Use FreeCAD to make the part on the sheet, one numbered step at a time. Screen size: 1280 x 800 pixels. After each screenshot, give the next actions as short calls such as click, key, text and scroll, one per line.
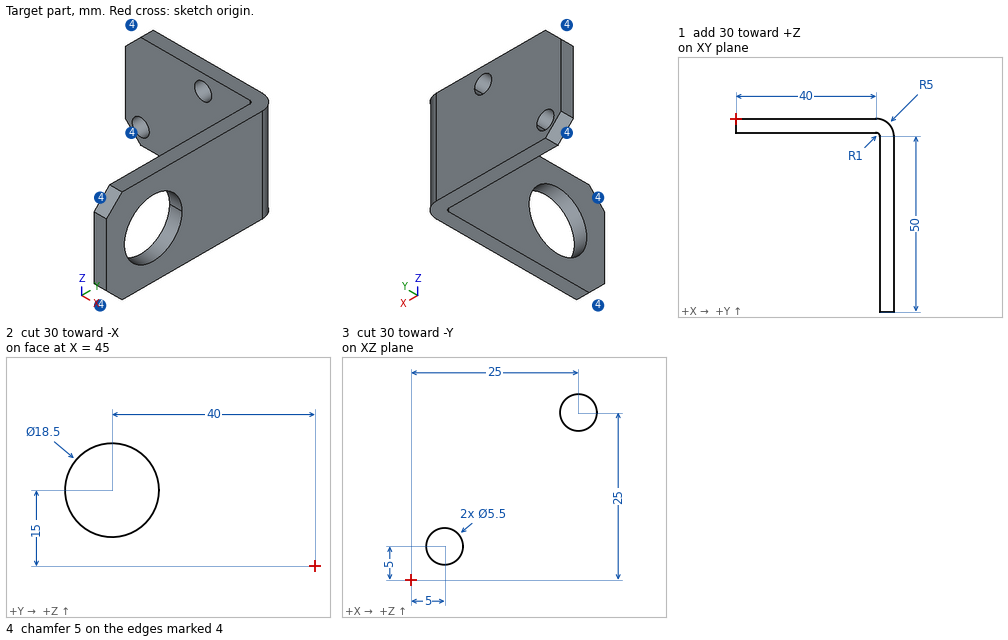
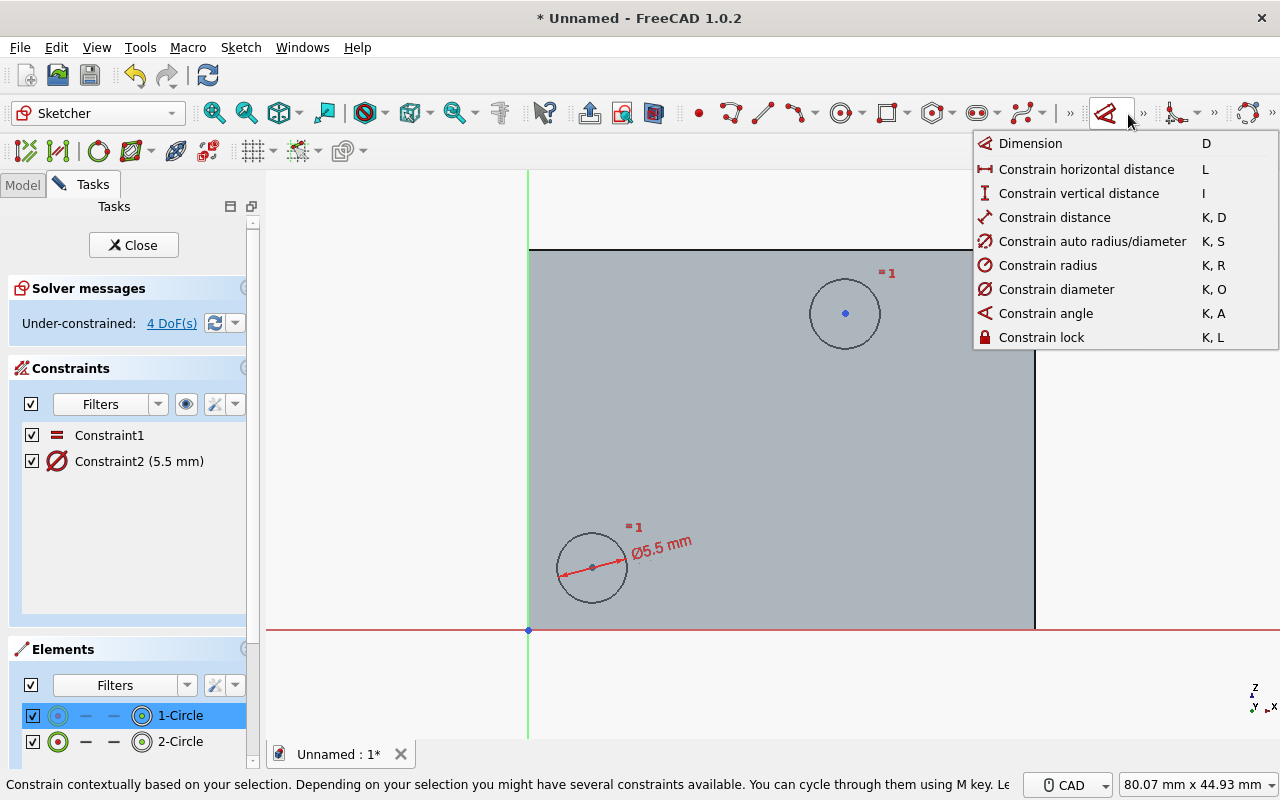
click(1126, 169)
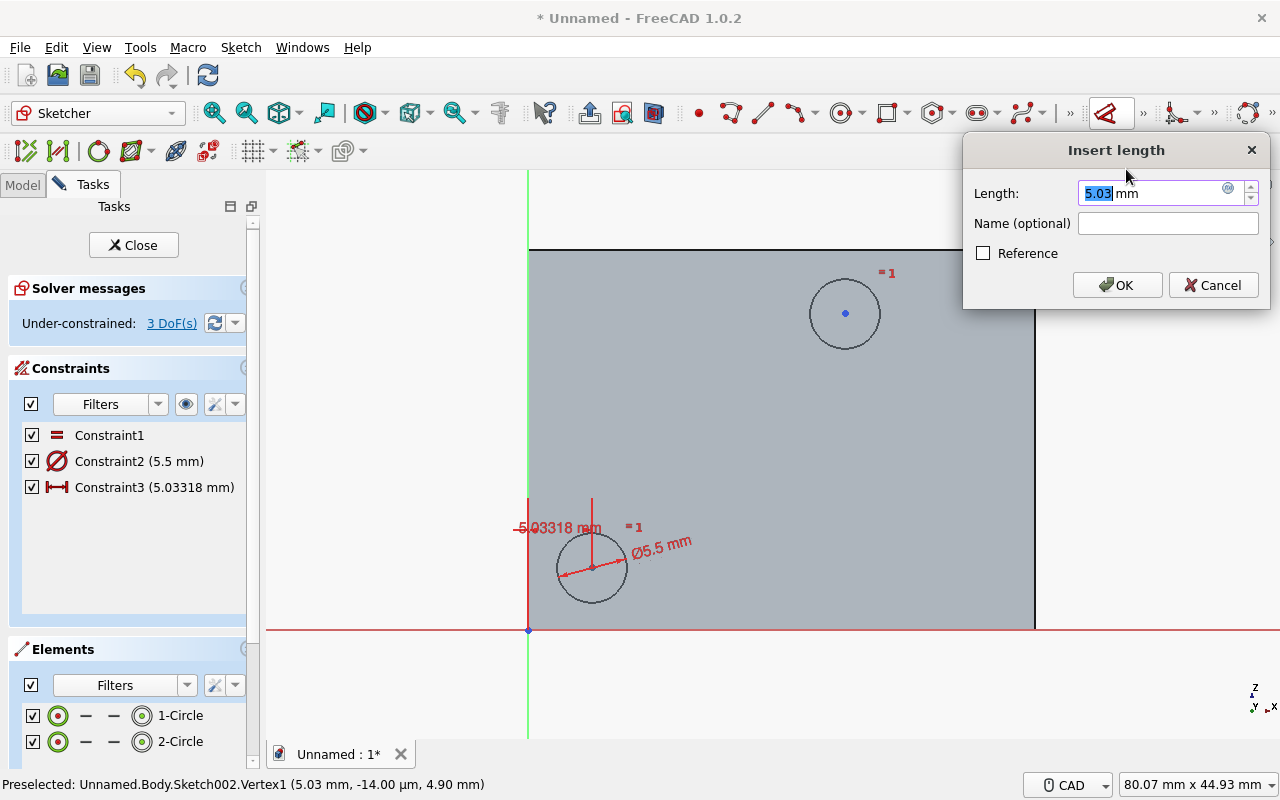
text(5)
key(Return)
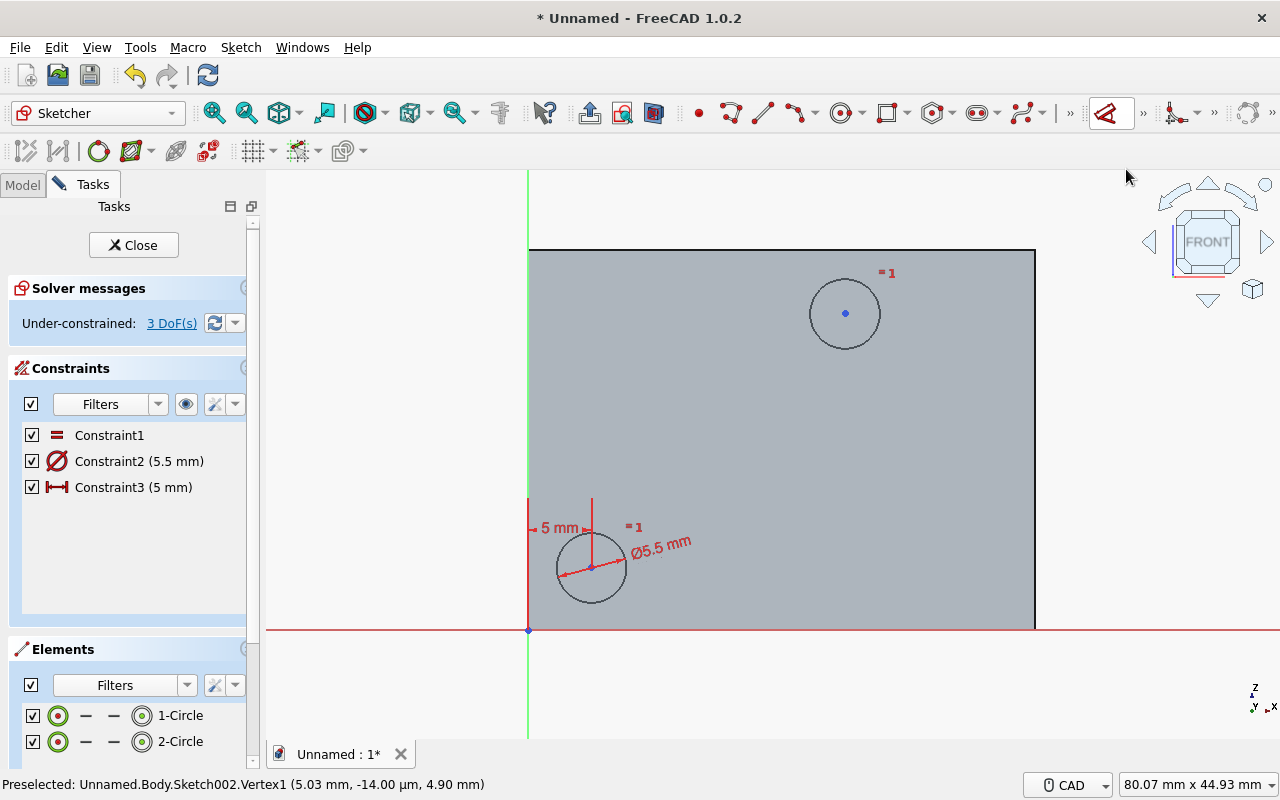
click(592, 568)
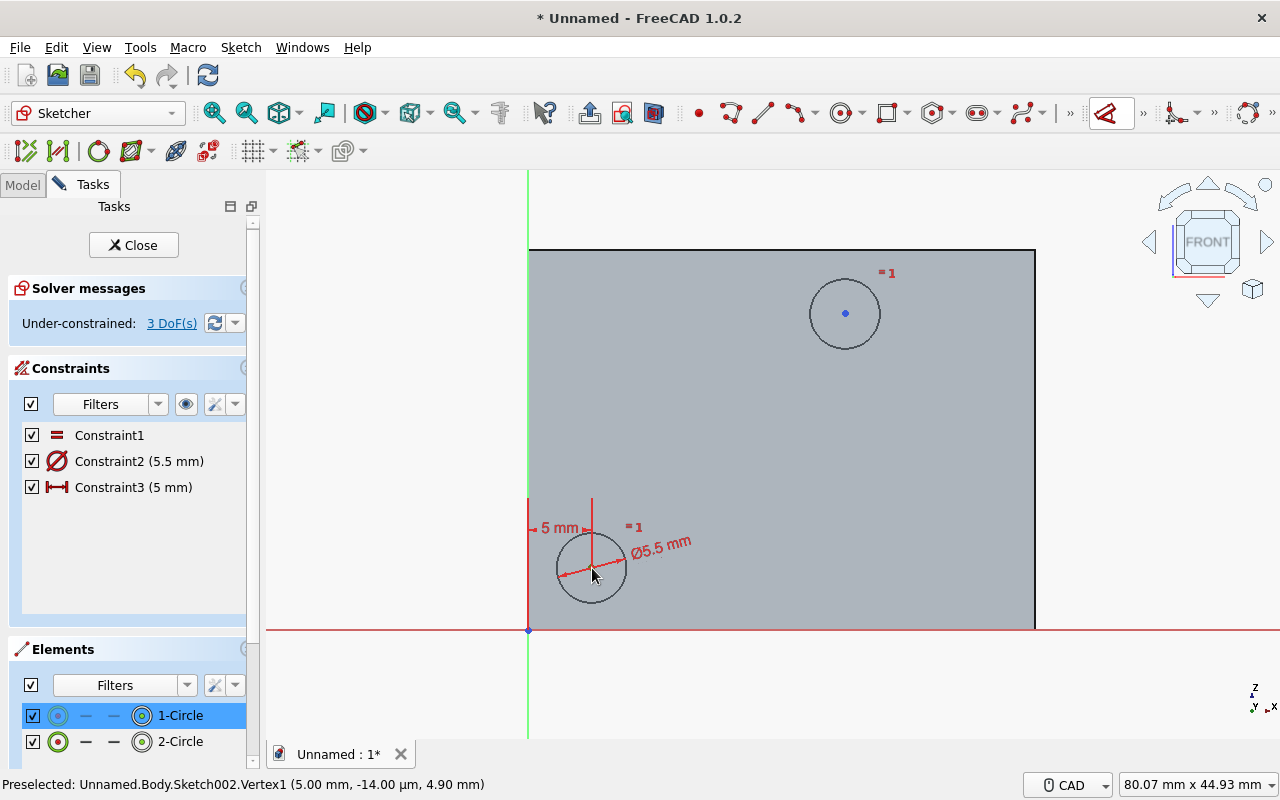
key(i)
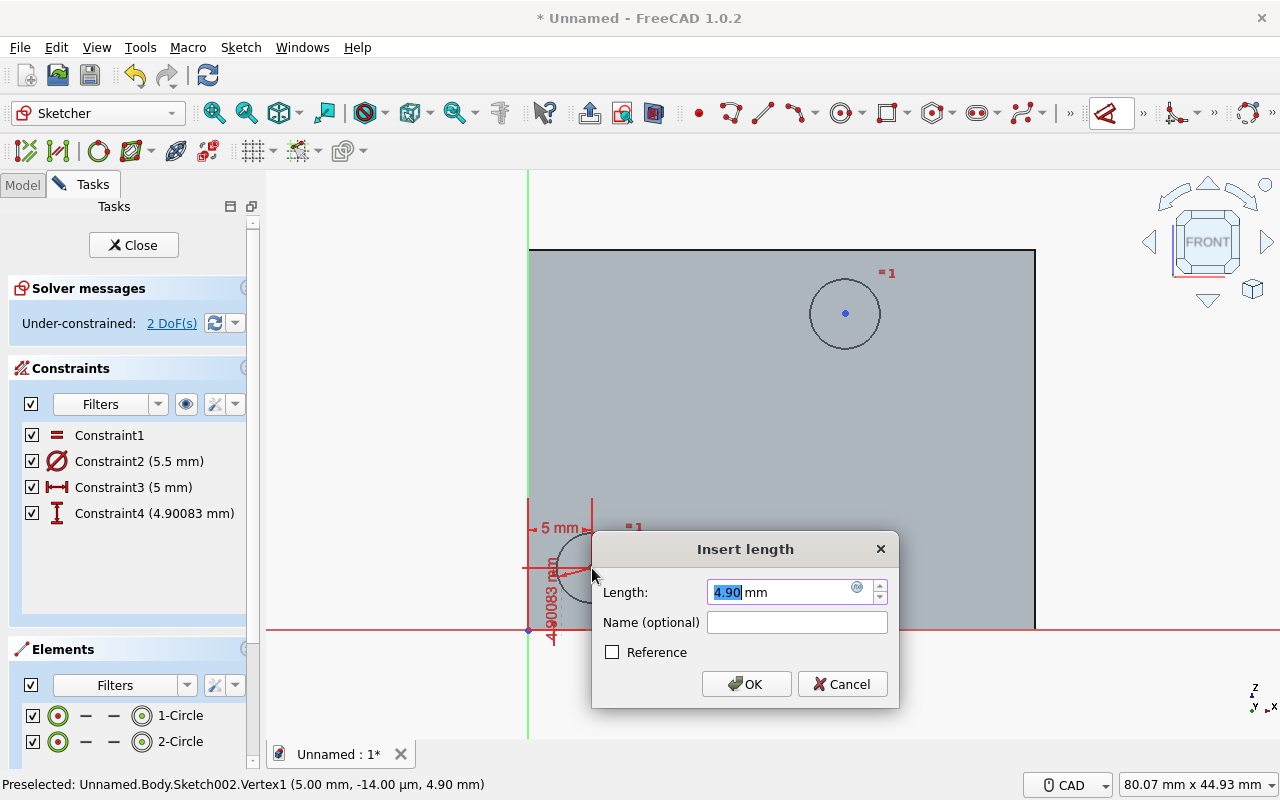
text(5)
key(Return)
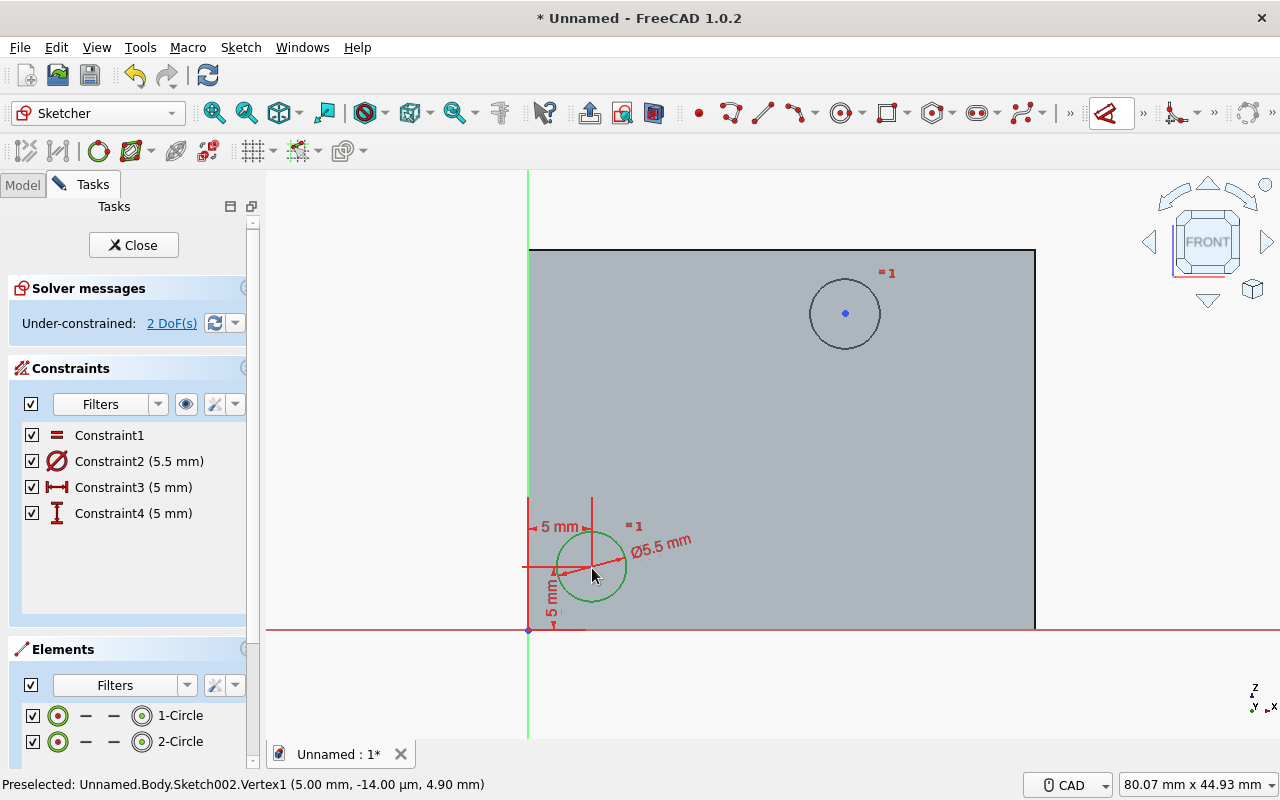
click(845, 314)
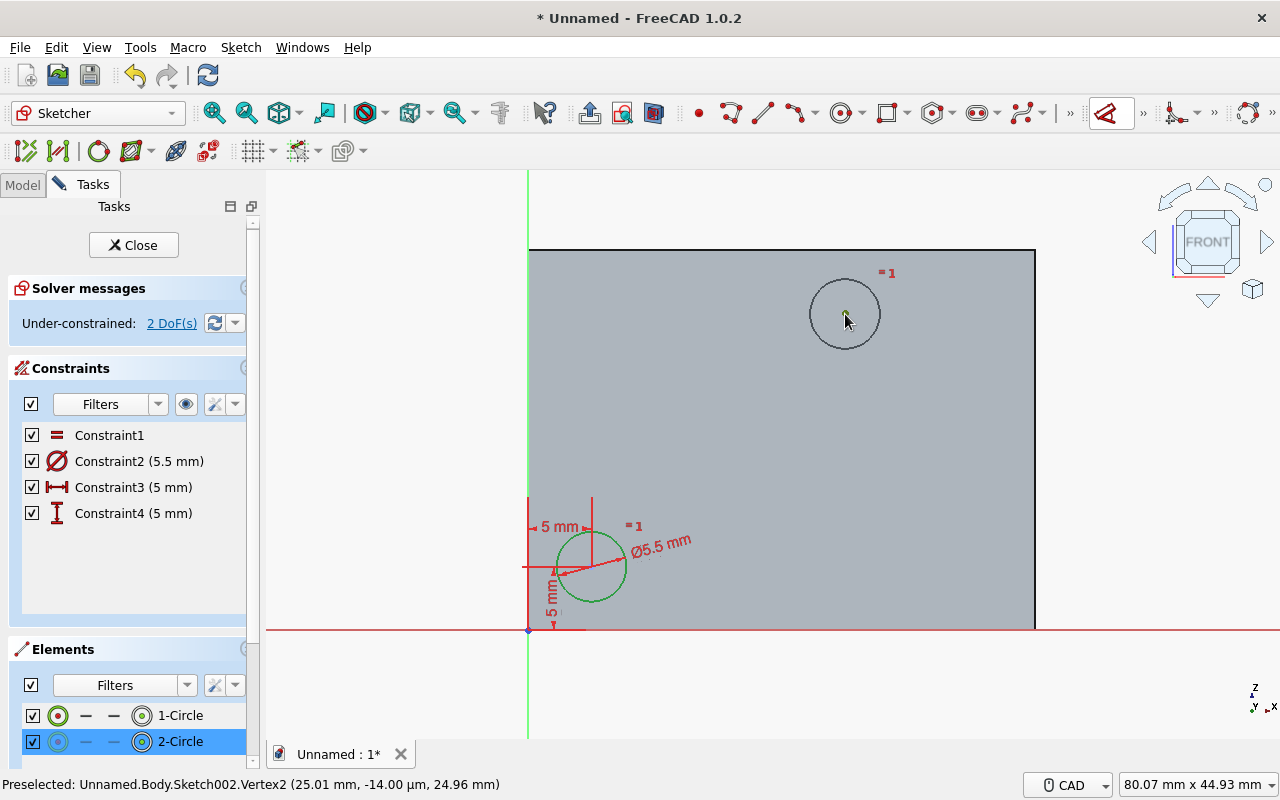
key(l)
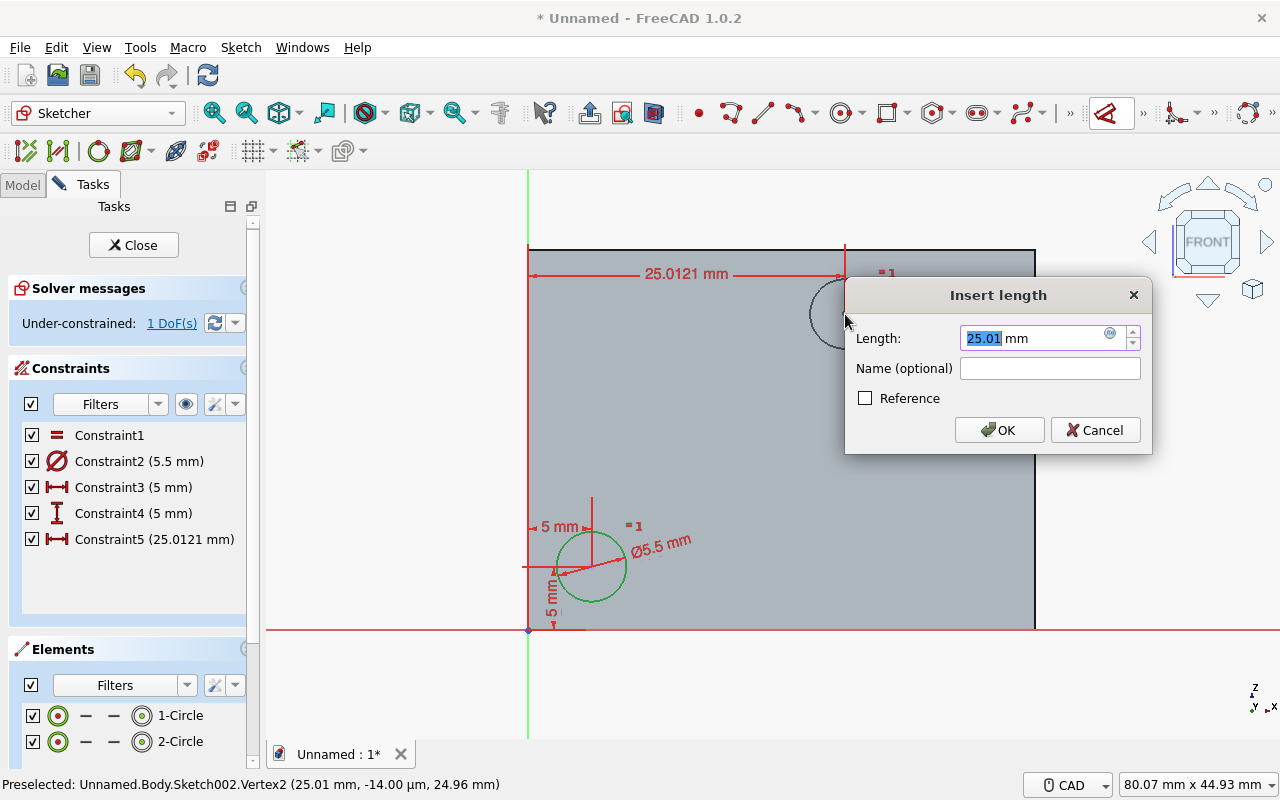
text(25)
key(Return)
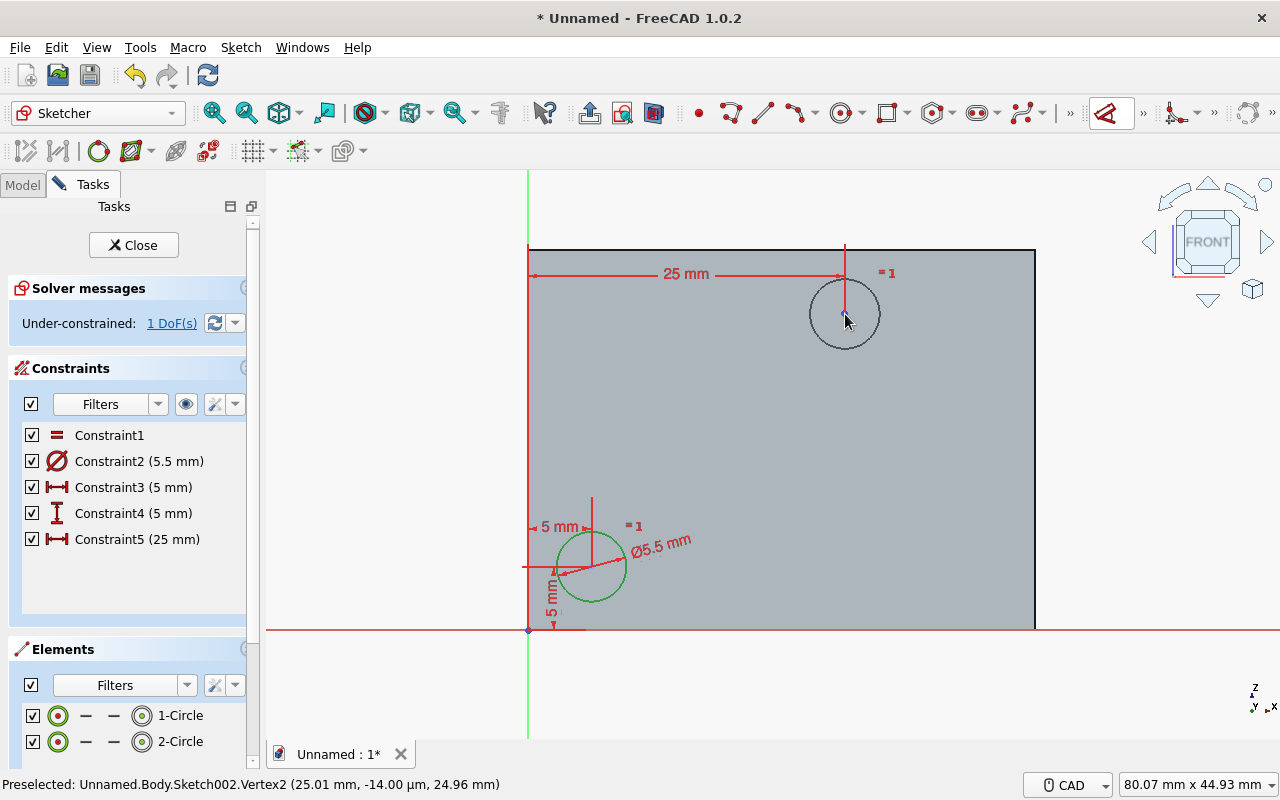
click(845, 314)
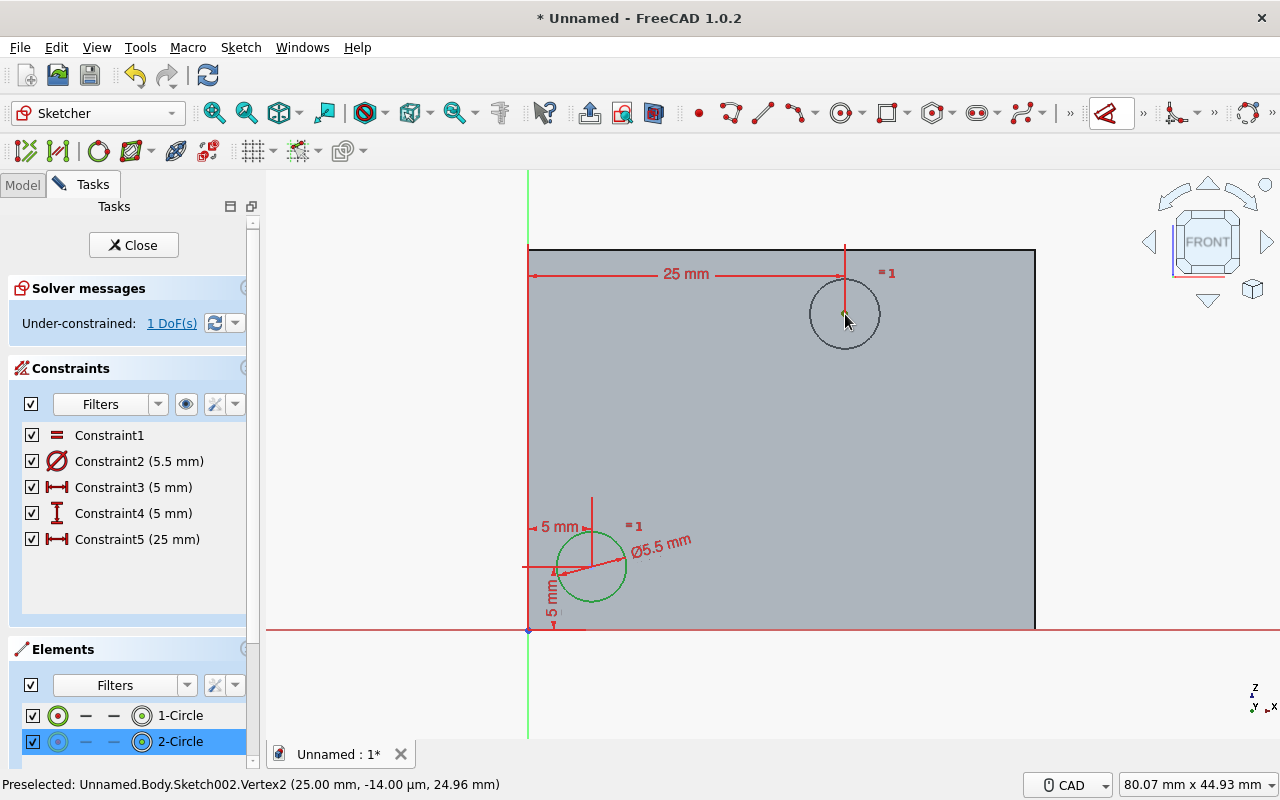
click(1128, 114)